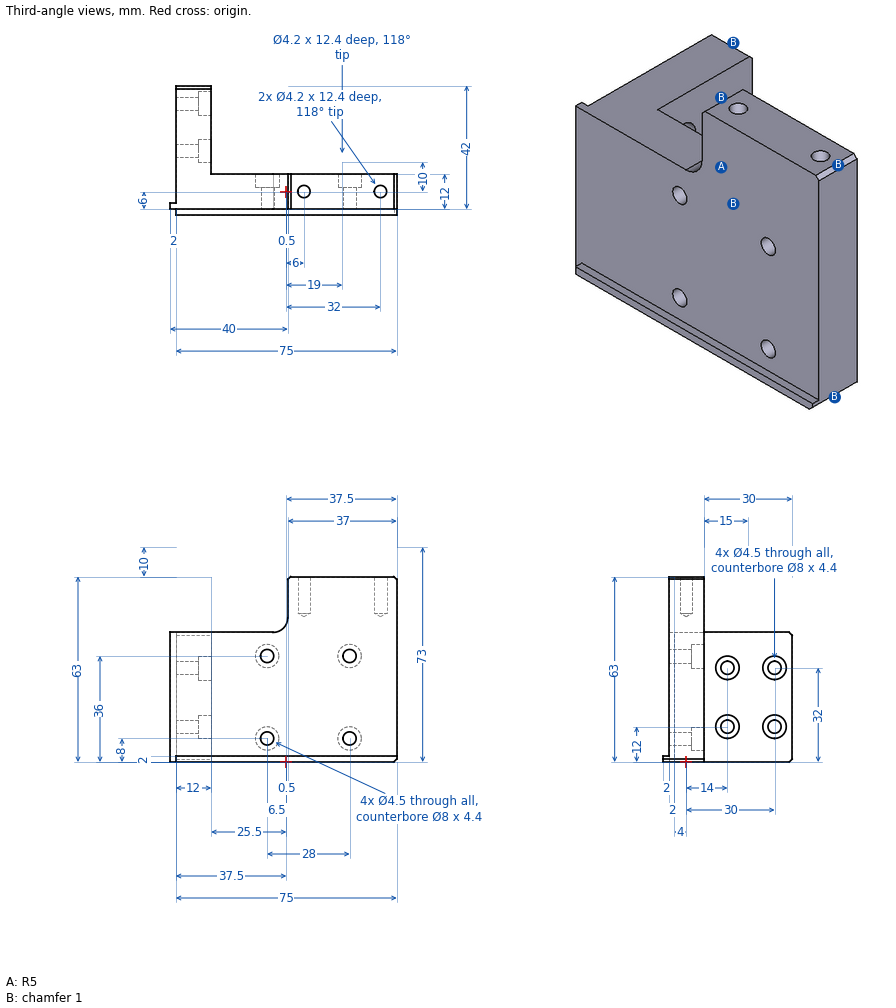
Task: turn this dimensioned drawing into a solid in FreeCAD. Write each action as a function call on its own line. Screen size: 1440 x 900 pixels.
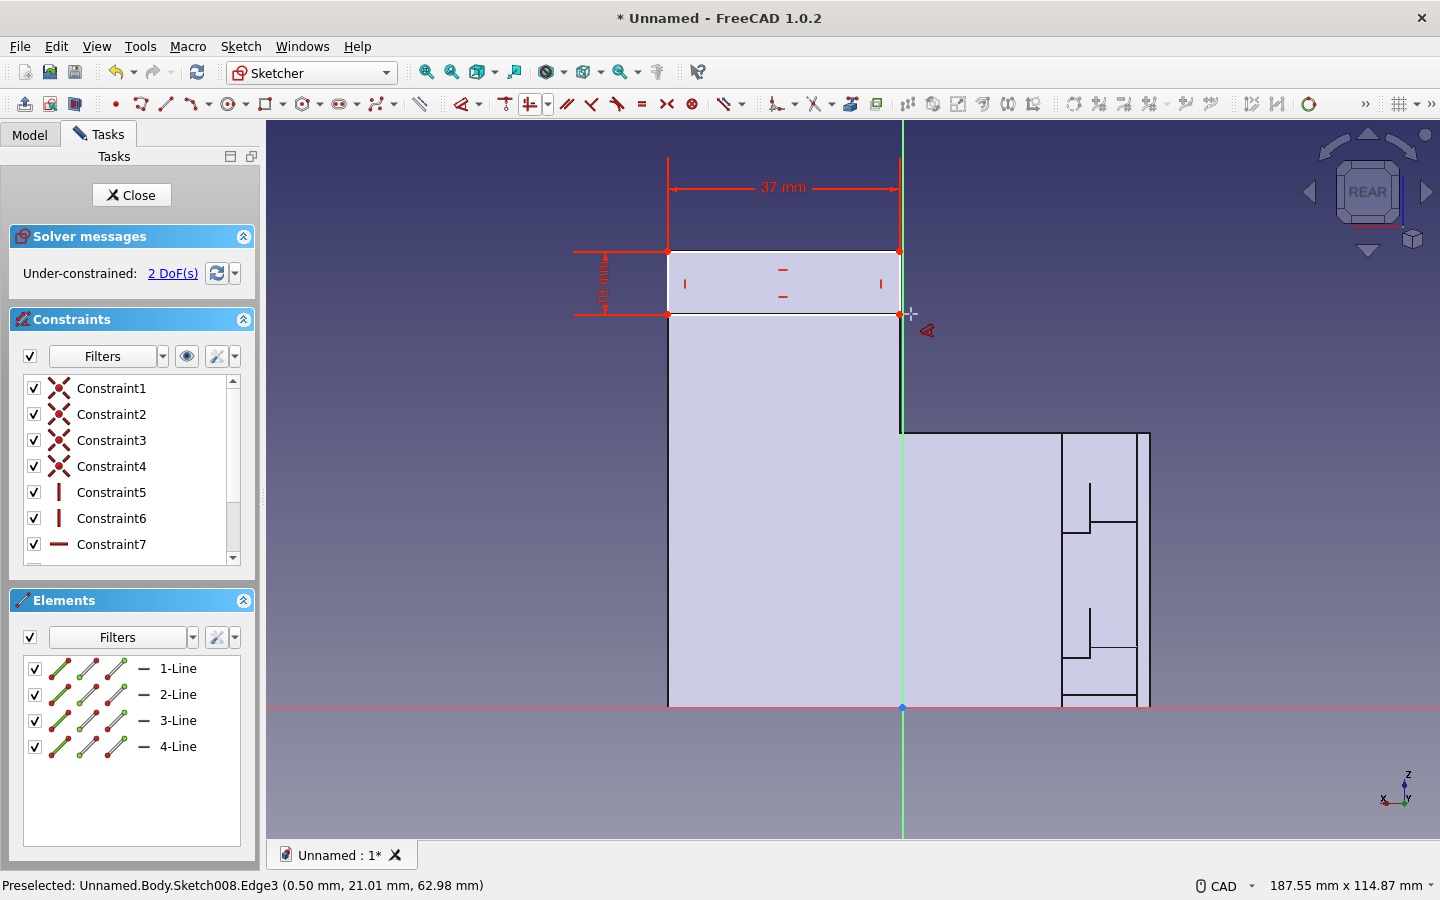
click(668, 252)
click(634, 480)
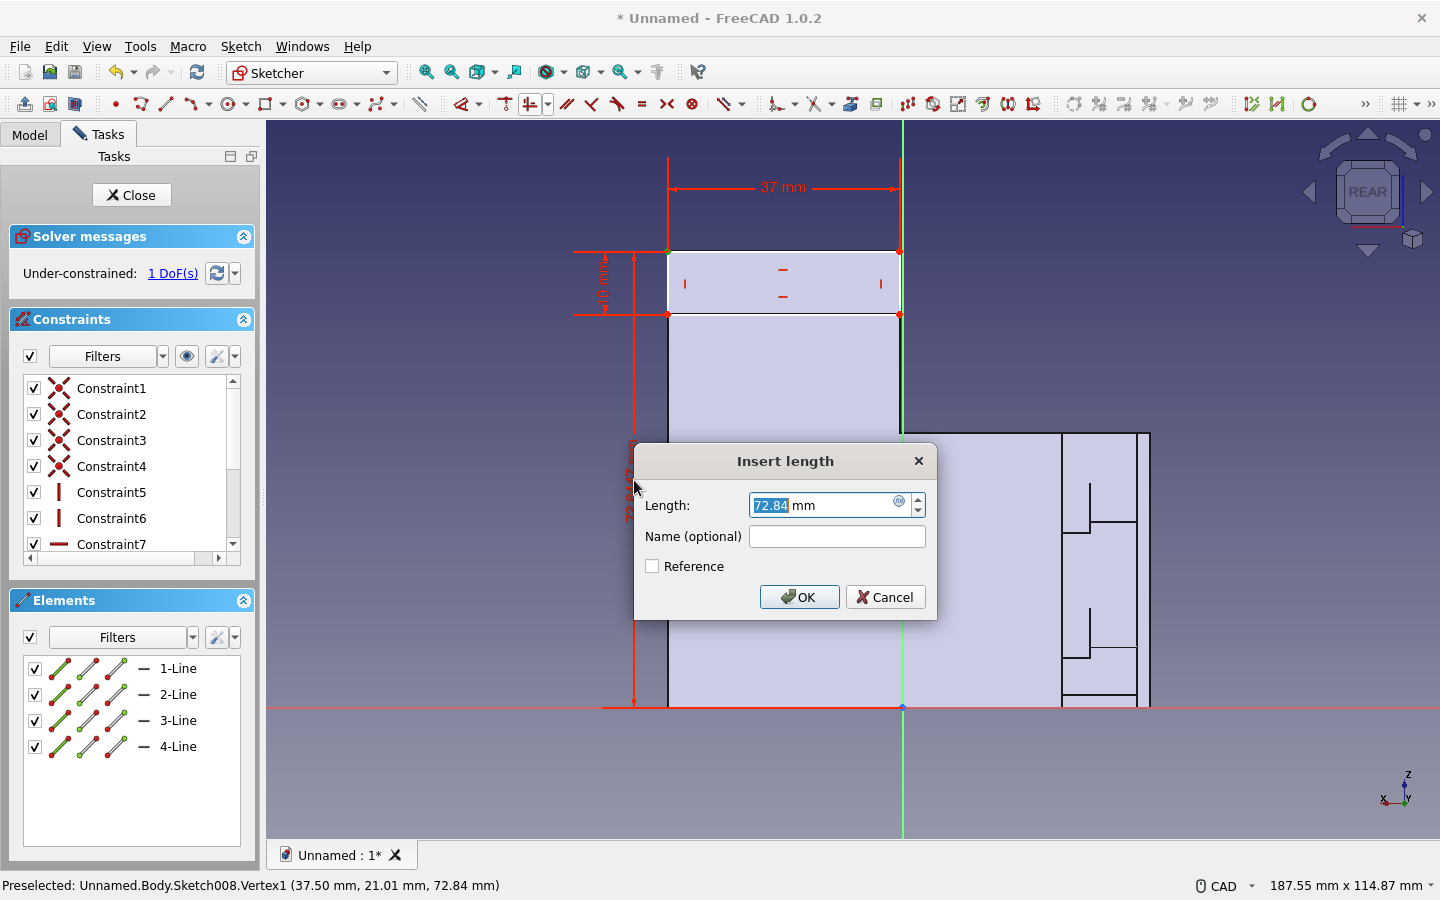
text(73)
key(Return)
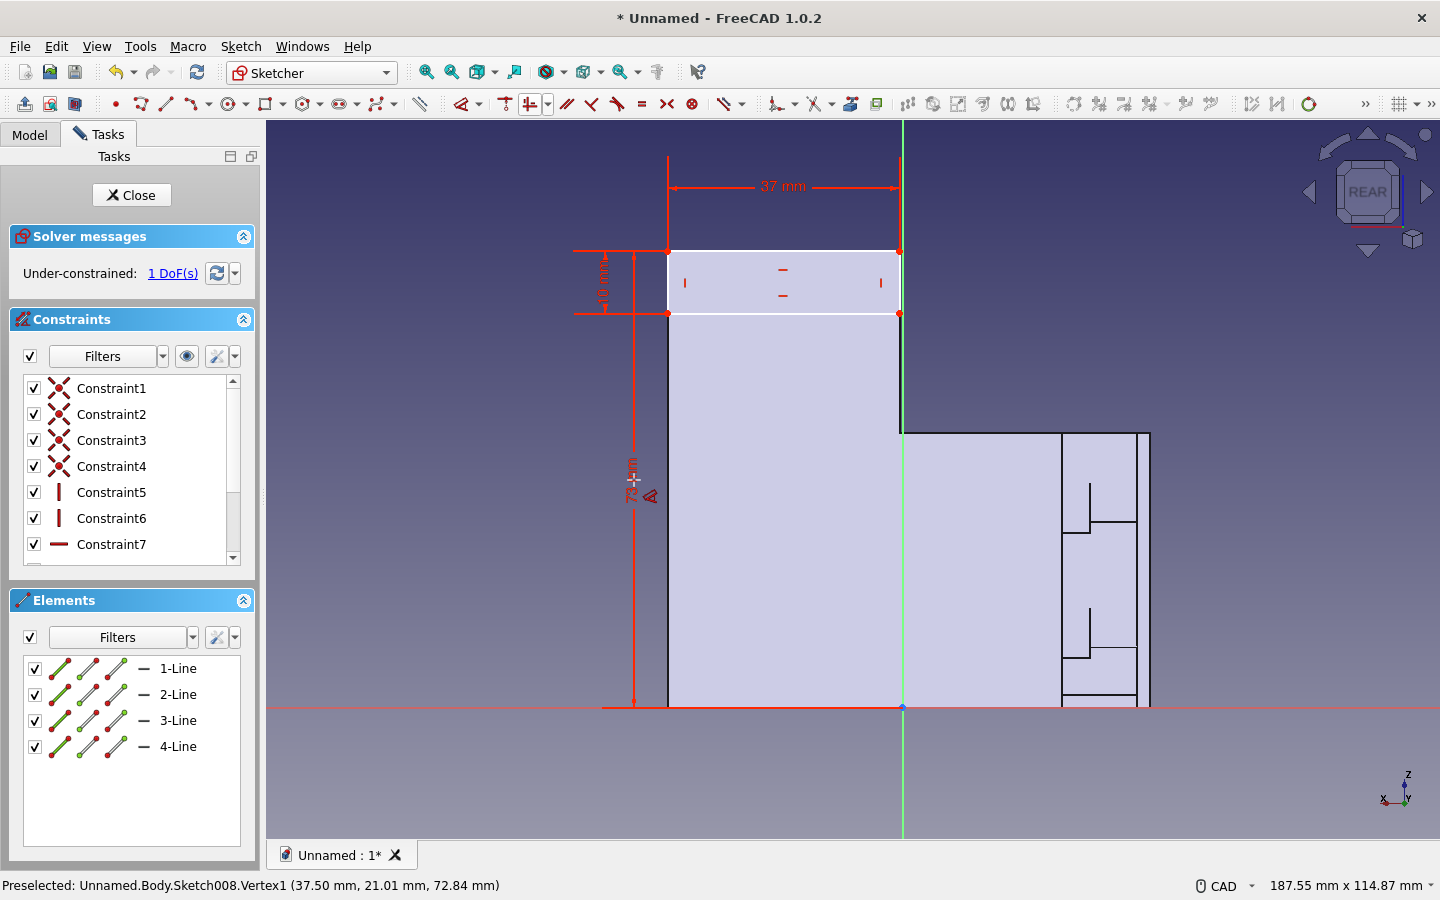
scroll(900, 314, up, 13)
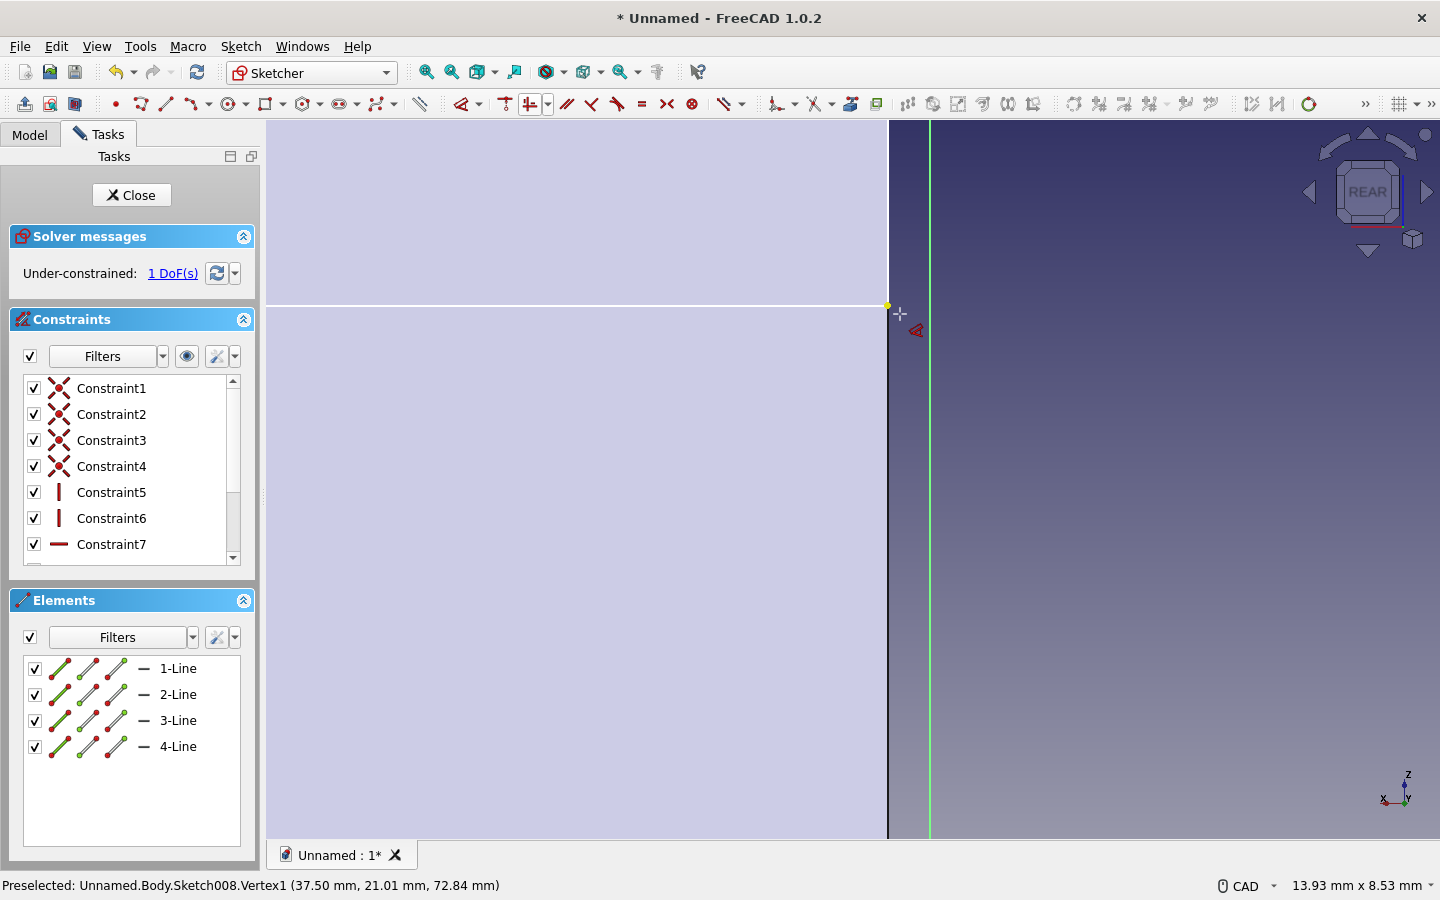
click(888, 306)
click(909, 272)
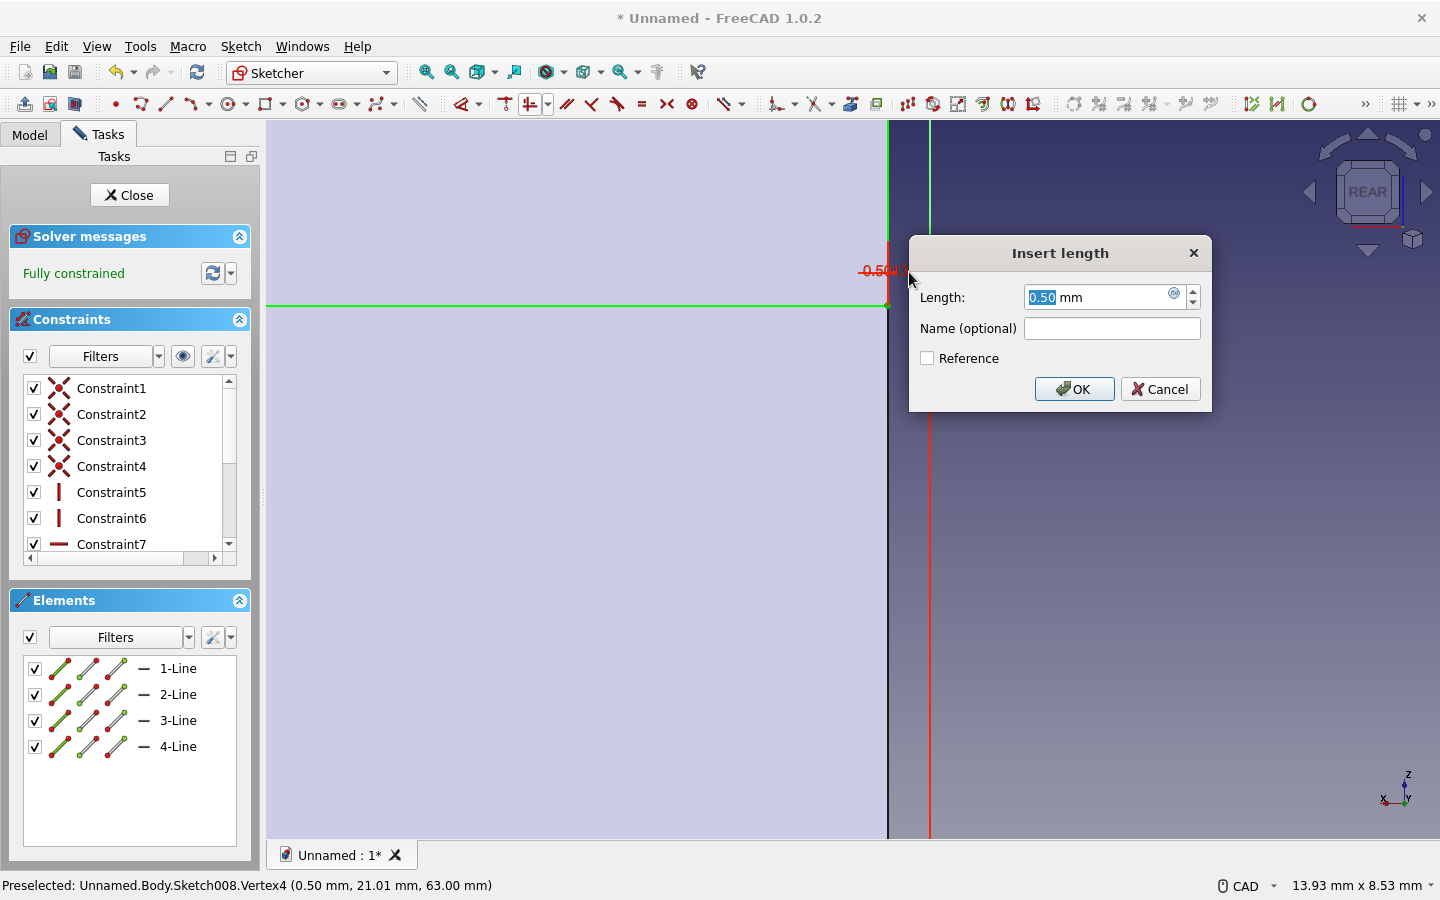
text(0.5)
key(Return)
key(Escape)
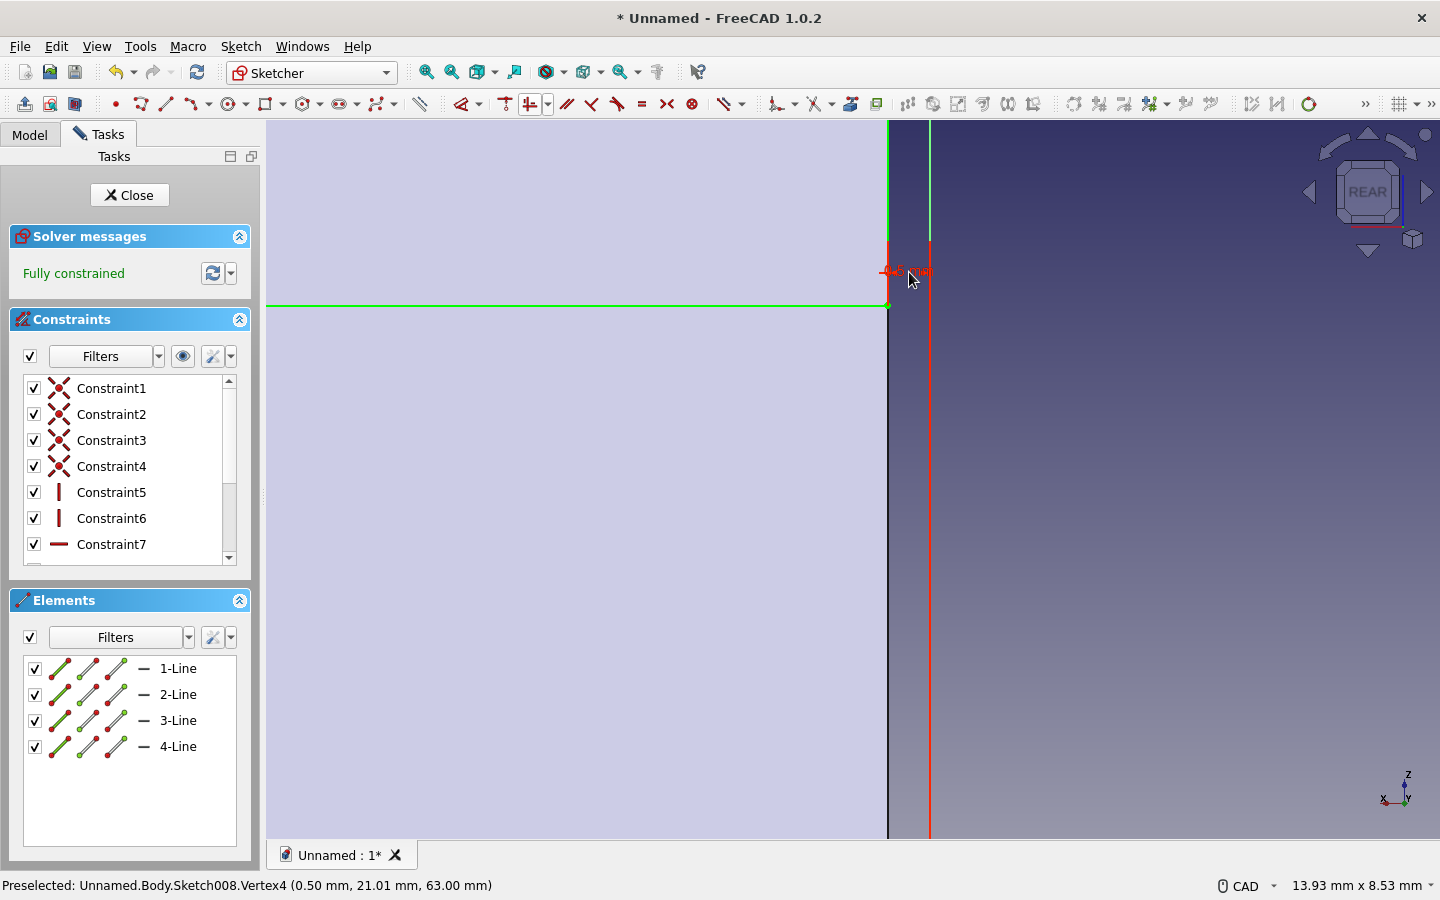
click(130, 195)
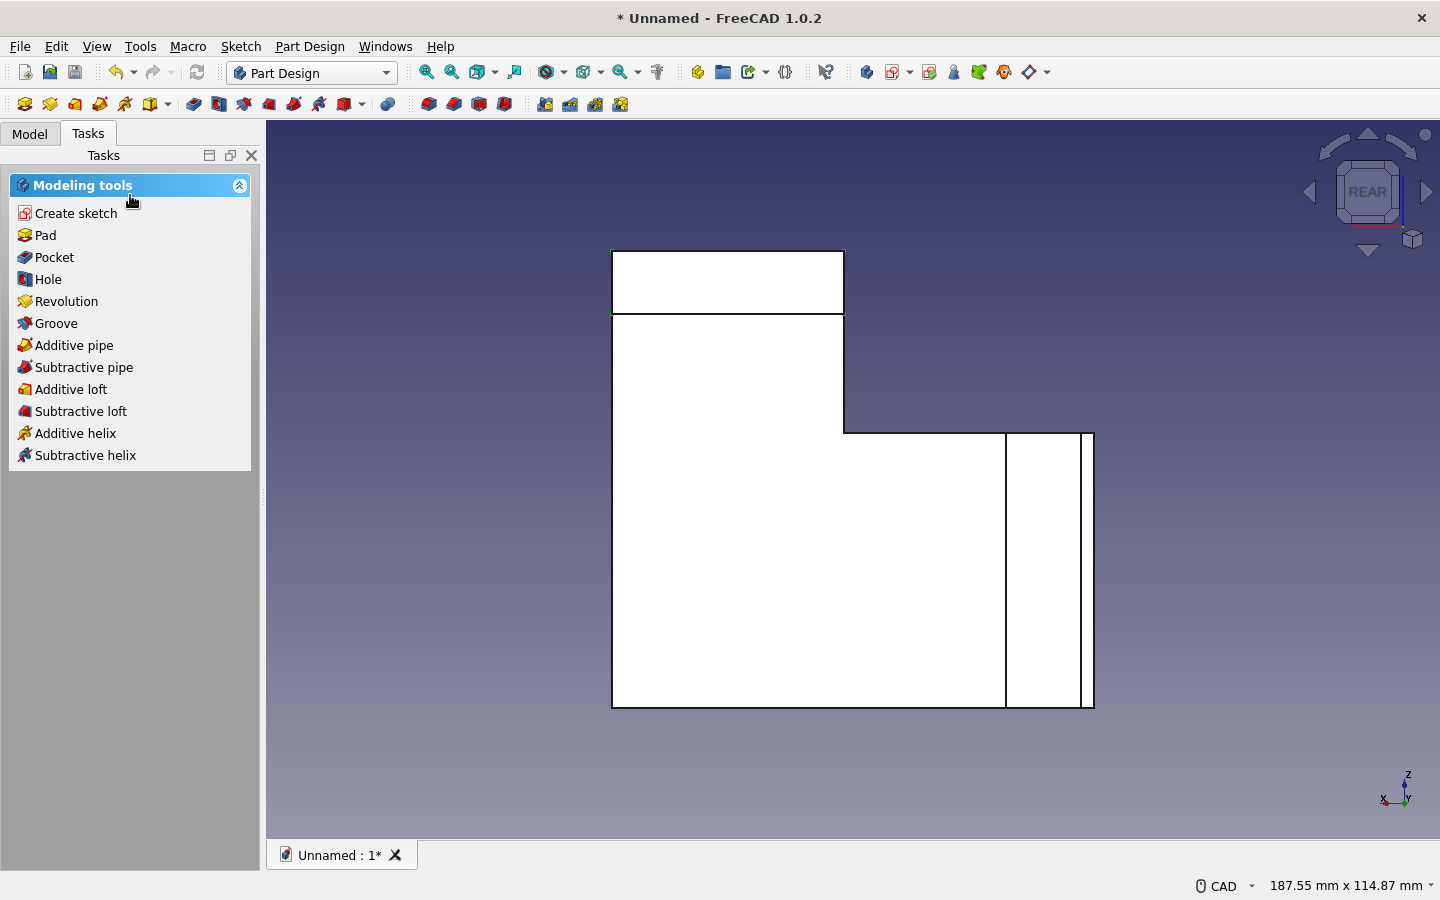
click(194, 104)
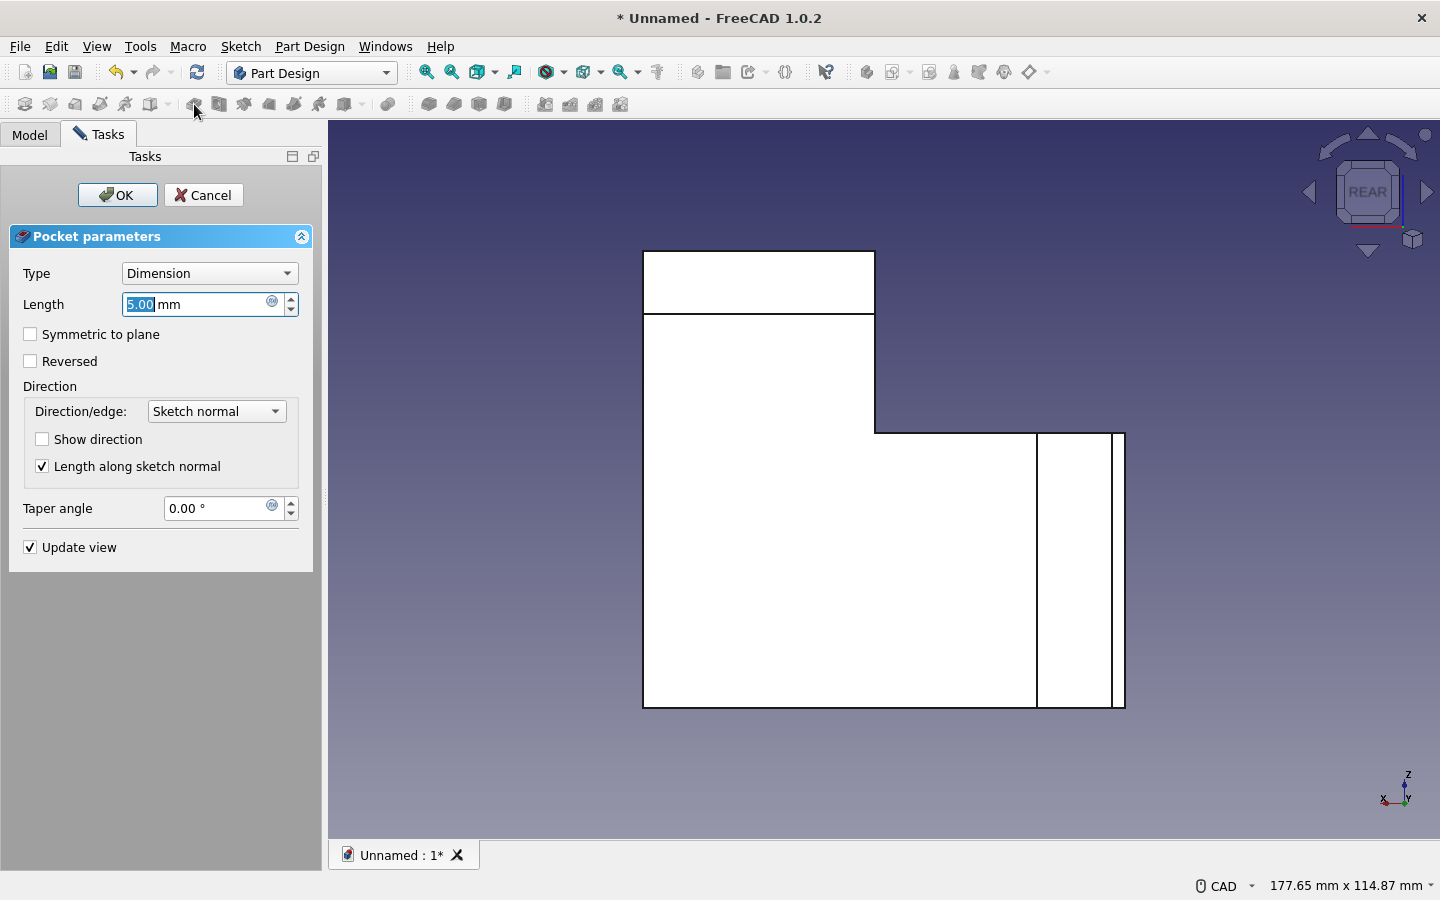
click(210, 274)